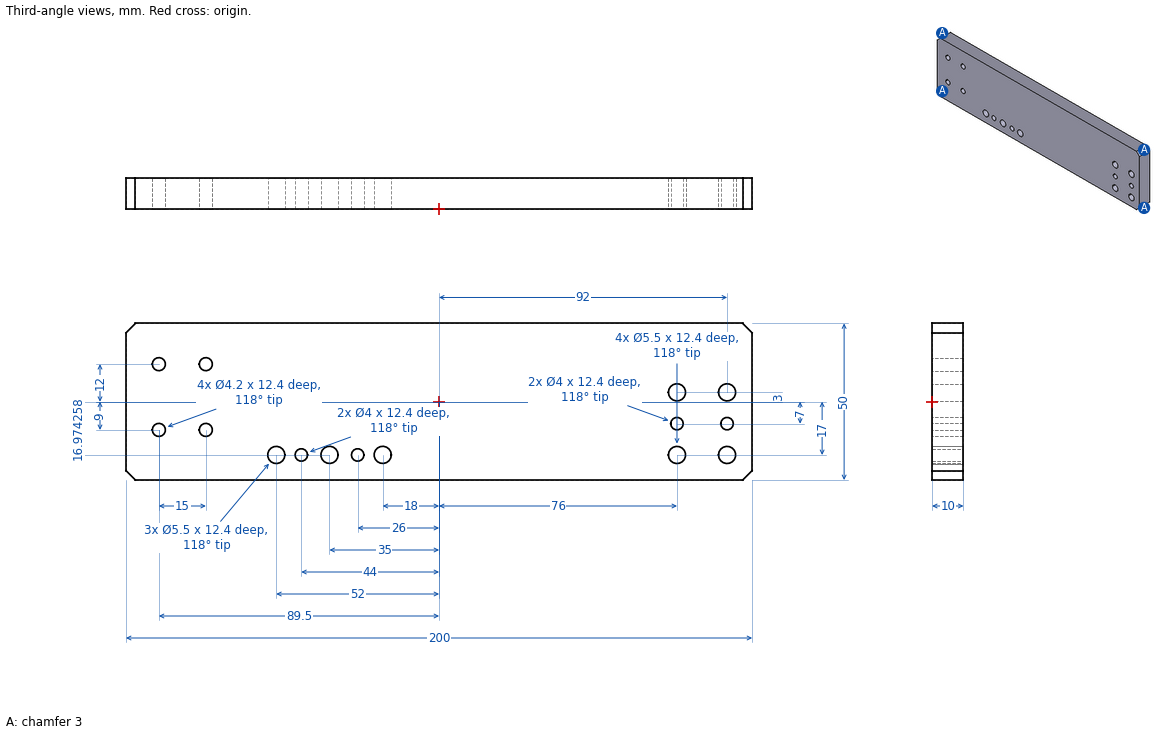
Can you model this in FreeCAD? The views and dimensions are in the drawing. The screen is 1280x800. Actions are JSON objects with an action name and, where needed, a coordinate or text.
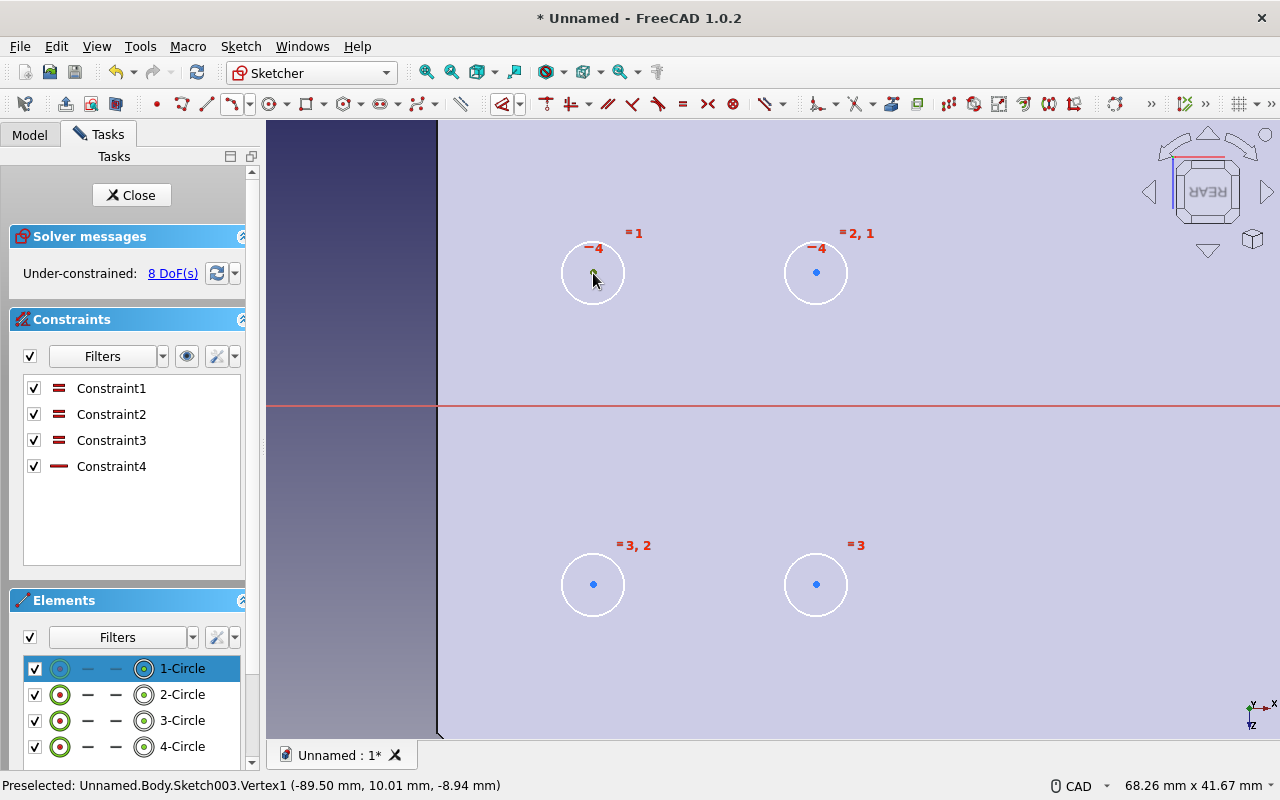
{"action": "left_click", "coordinate": [593, 585]}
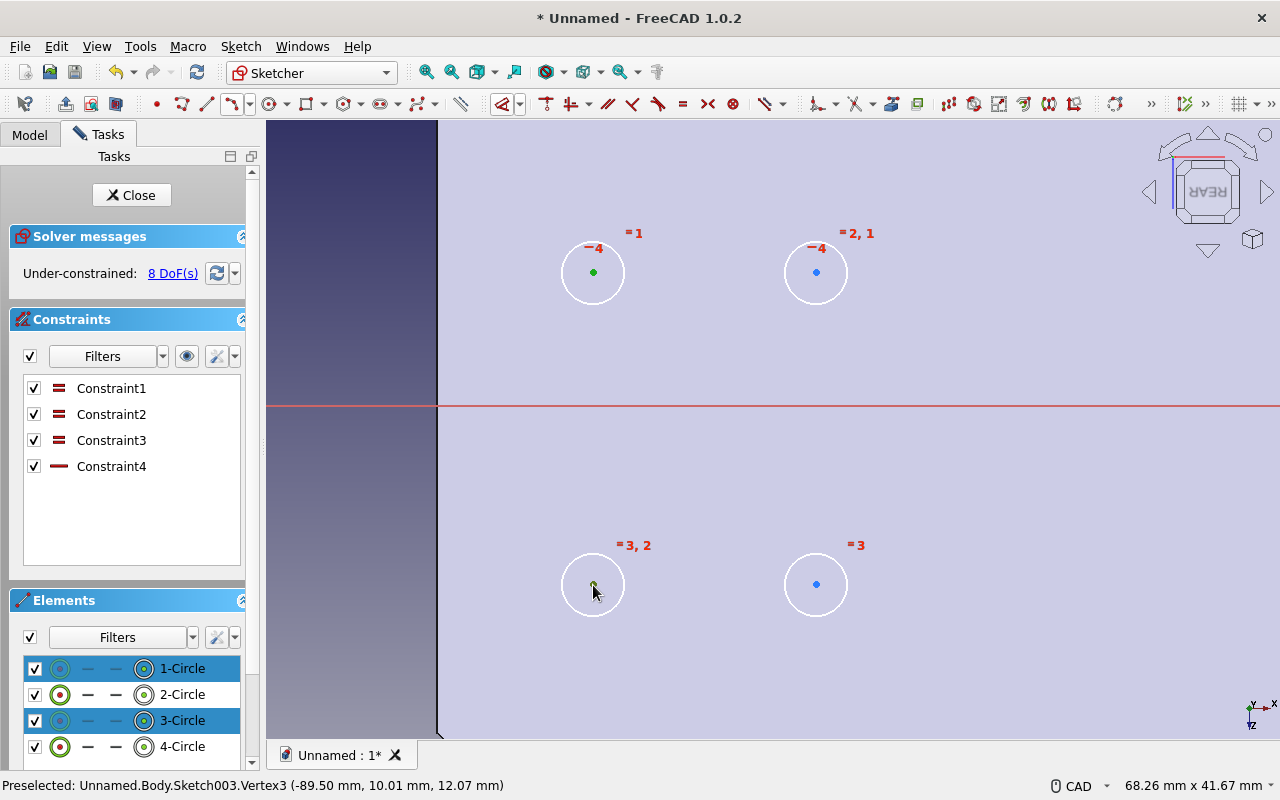
{"action": "key", "text": "v"}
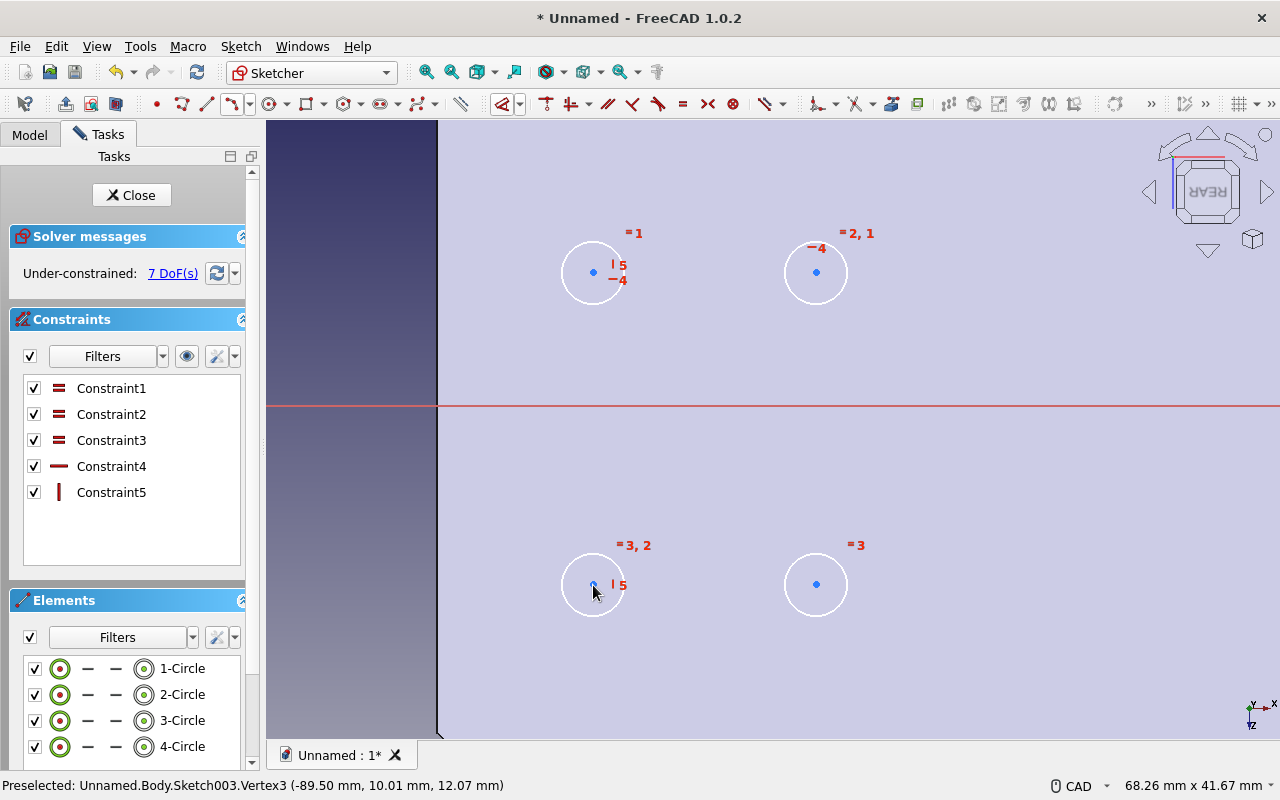
{"action": "left_click", "coordinate": [816, 273]}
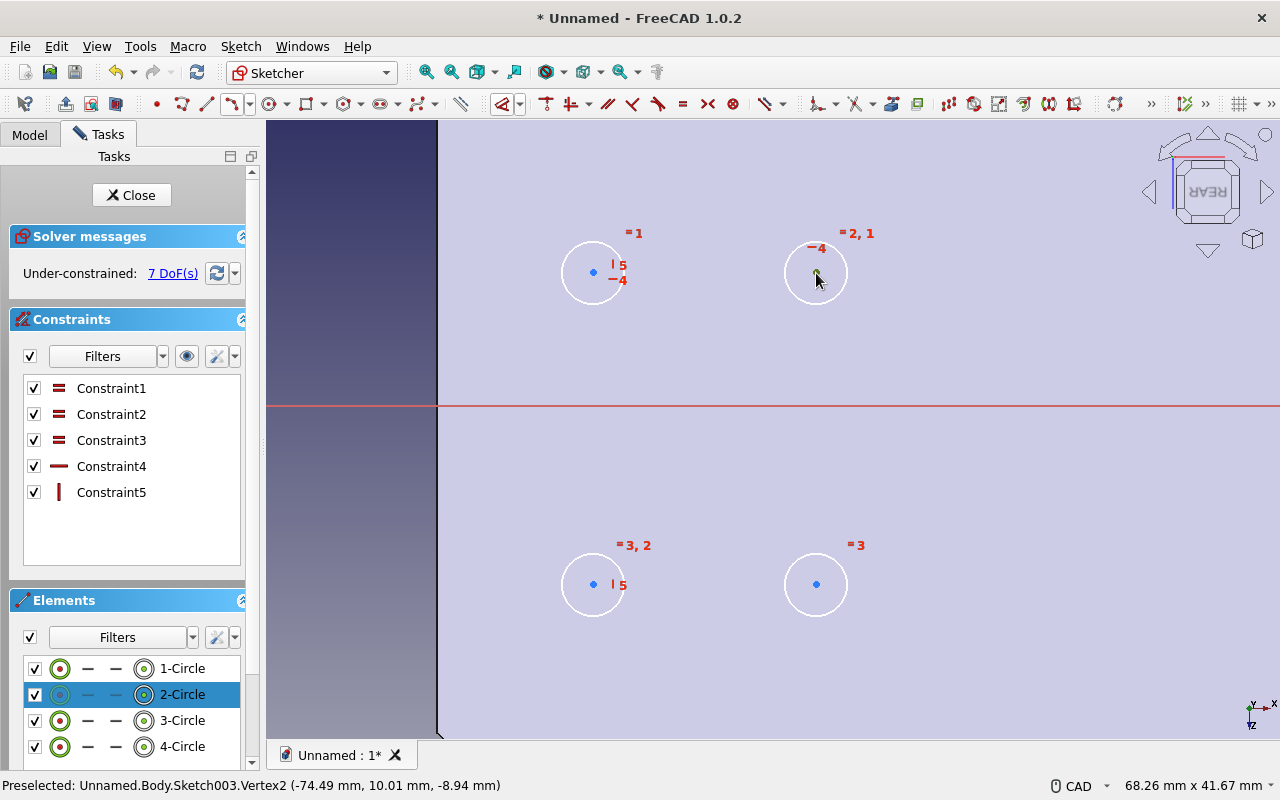
{"action": "left_click", "coordinate": [816, 585]}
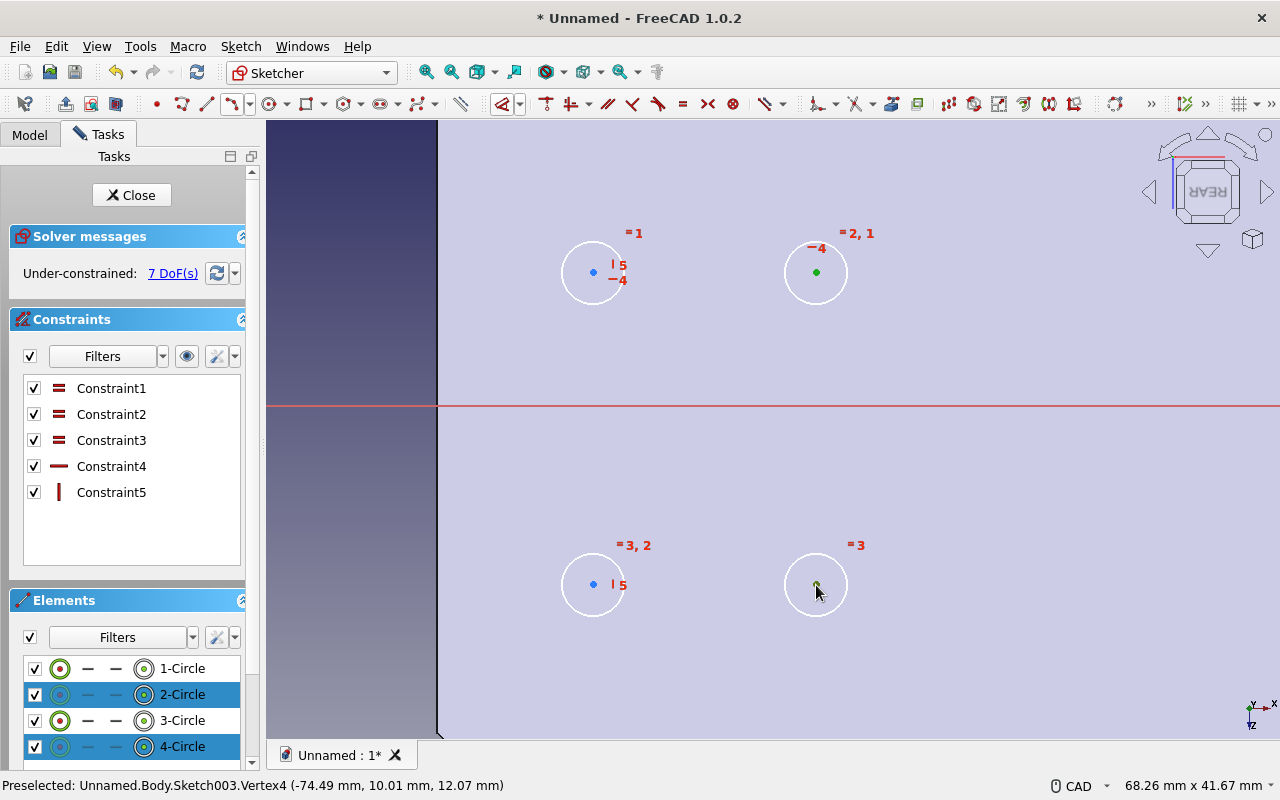
{"action": "left_click", "coordinate": [588, 104]}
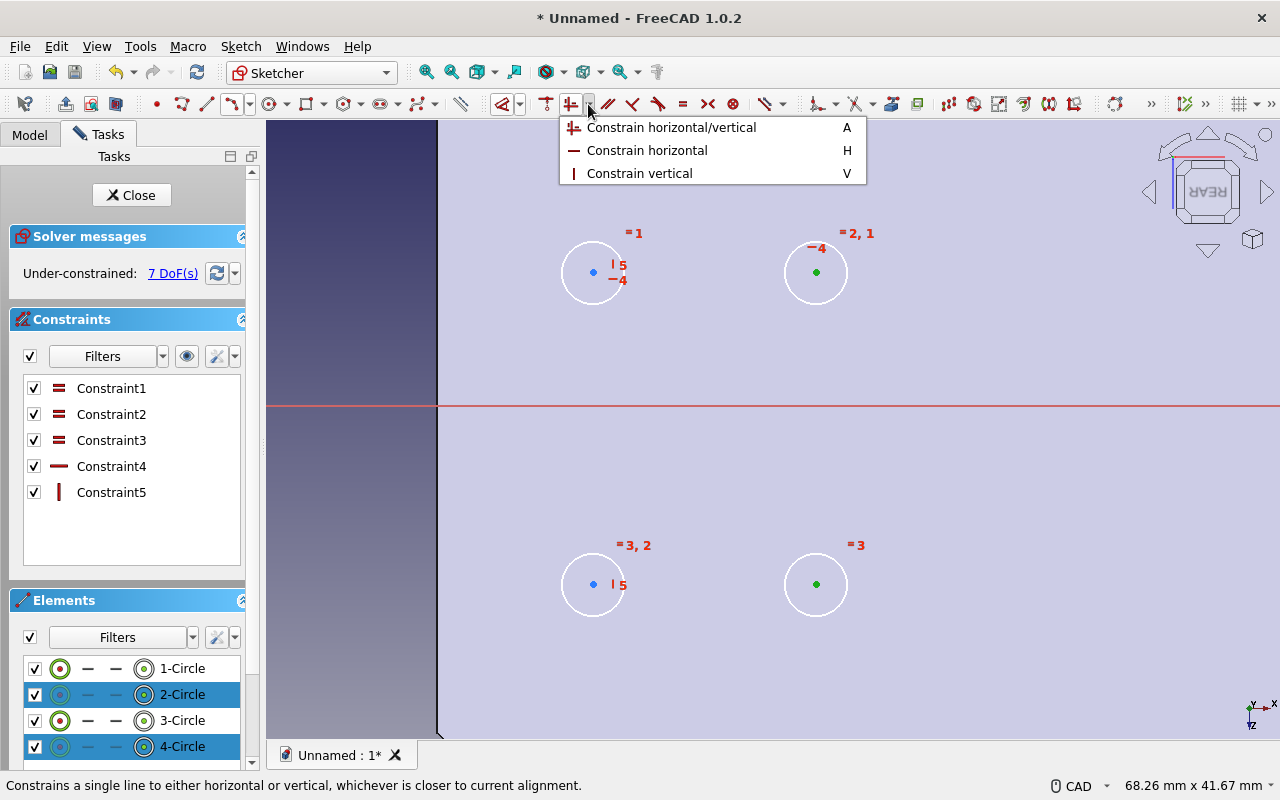
{"action": "left_click", "coordinate": [713, 174]}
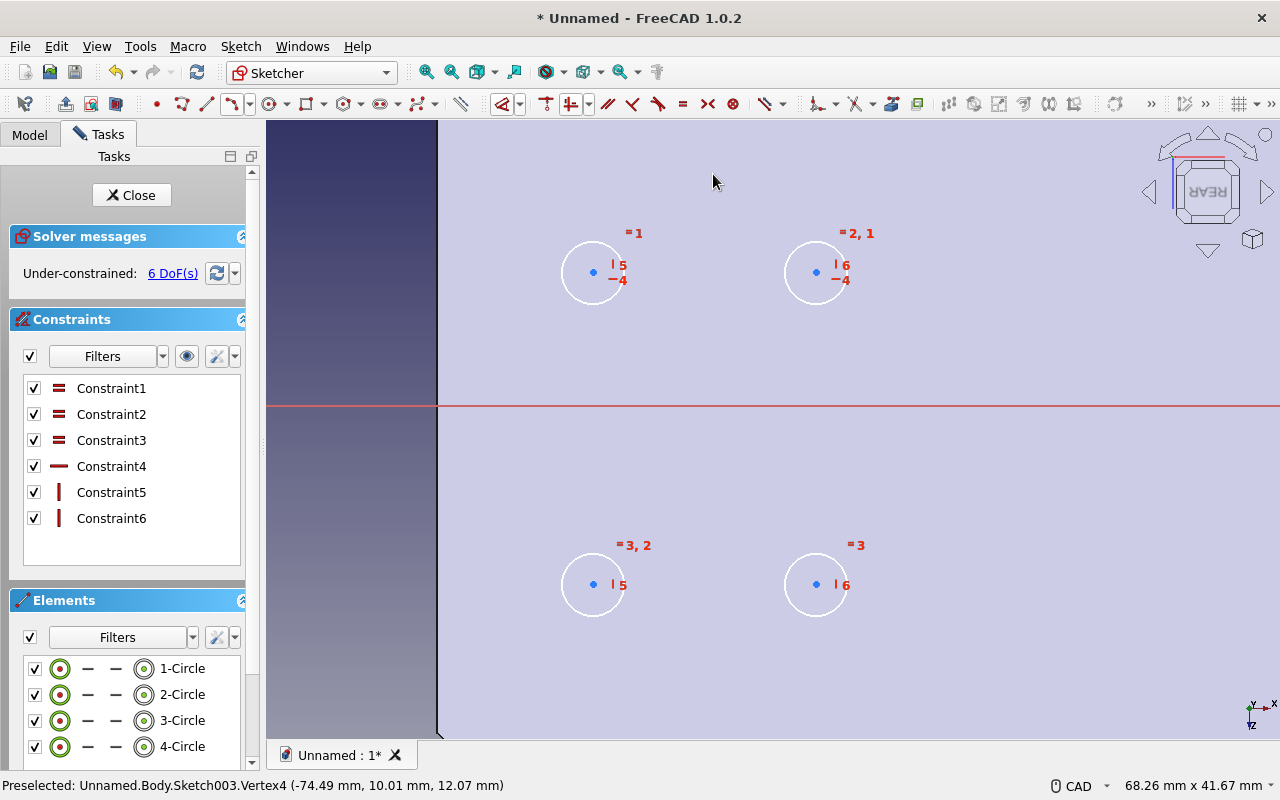
{"action": "left_click", "coordinate": [593, 585]}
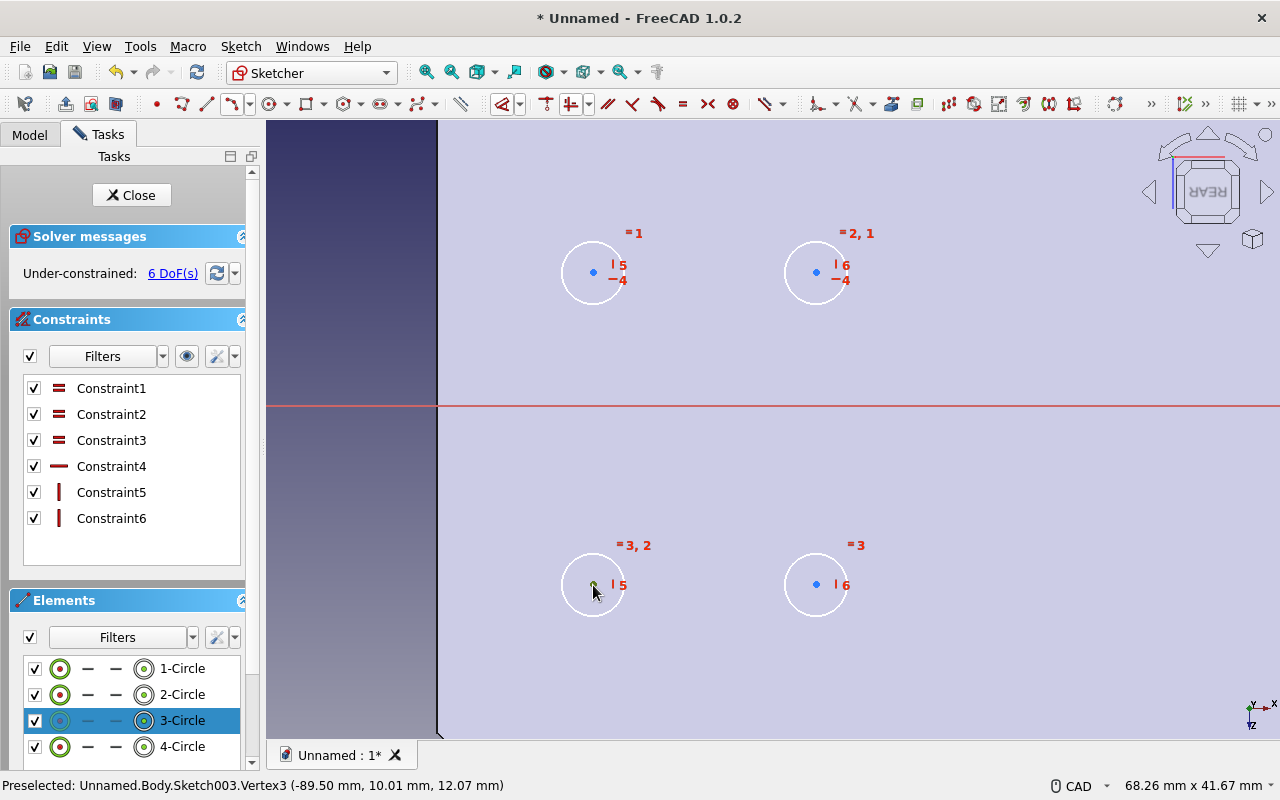
{"action": "left_click", "coordinate": [816, 585]}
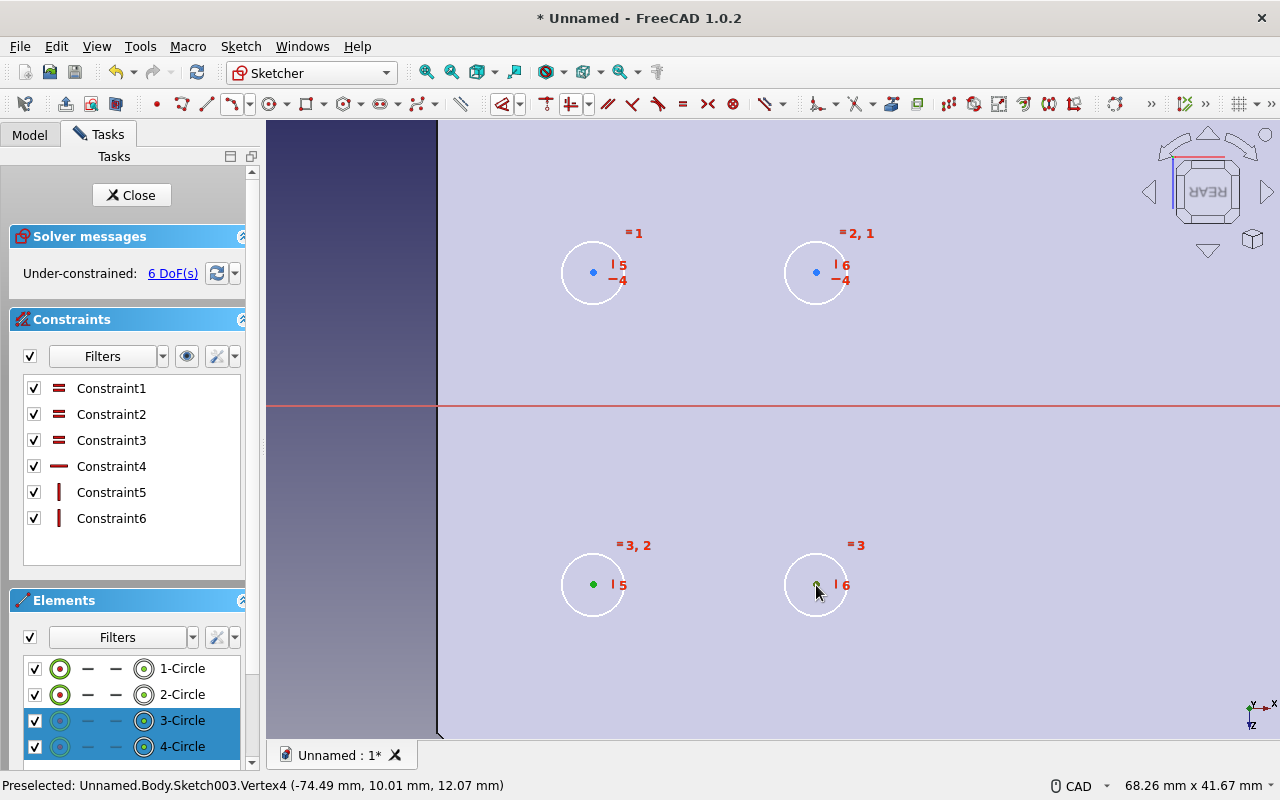
{"action": "left_click", "coordinate": [588, 104]}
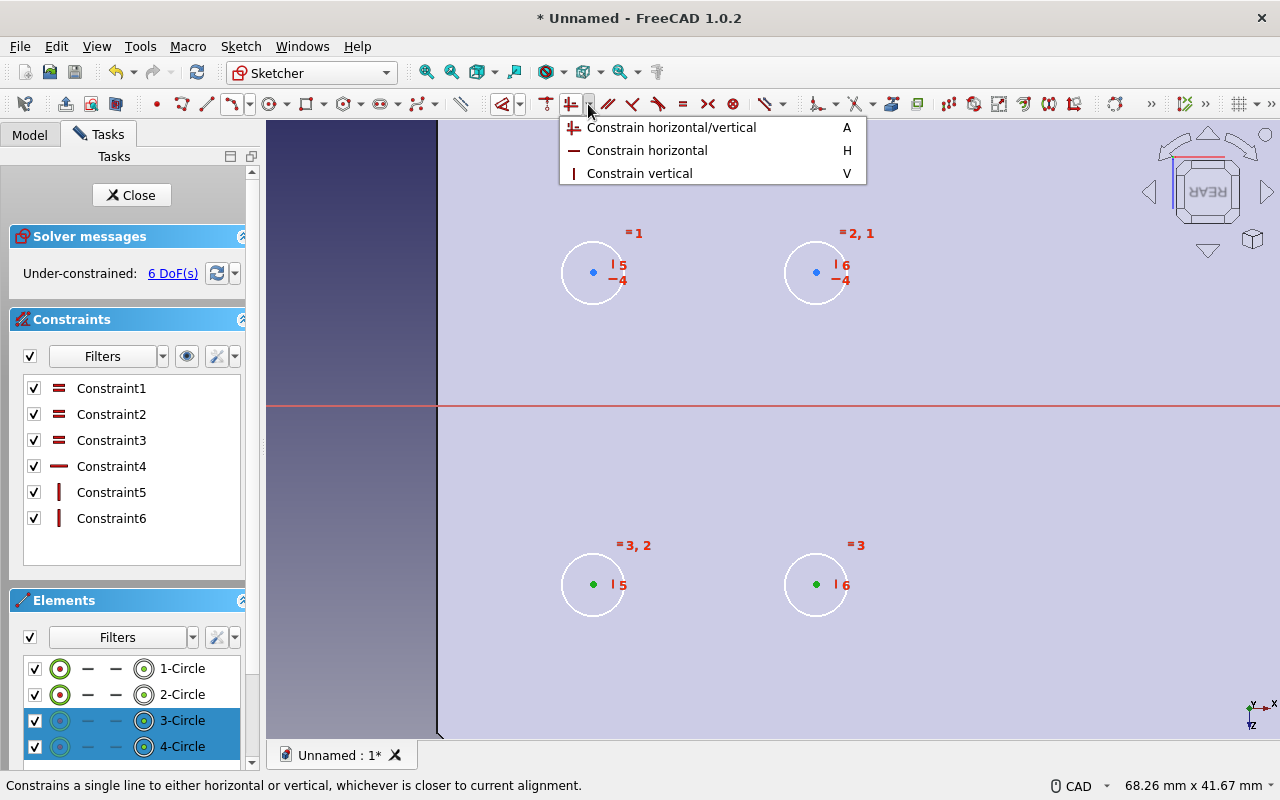
{"action": "left_click", "coordinate": [713, 150]}